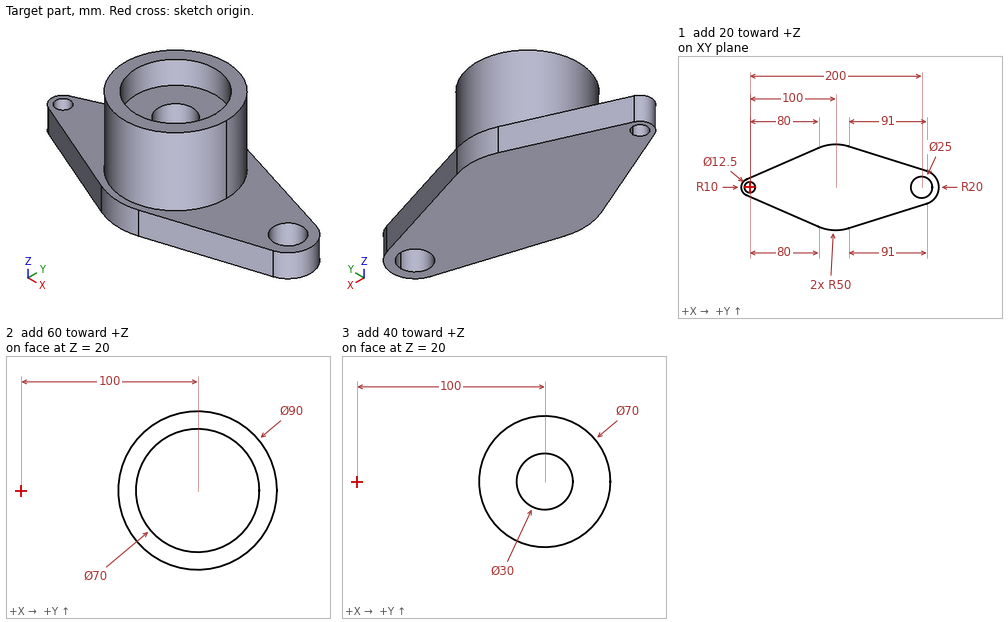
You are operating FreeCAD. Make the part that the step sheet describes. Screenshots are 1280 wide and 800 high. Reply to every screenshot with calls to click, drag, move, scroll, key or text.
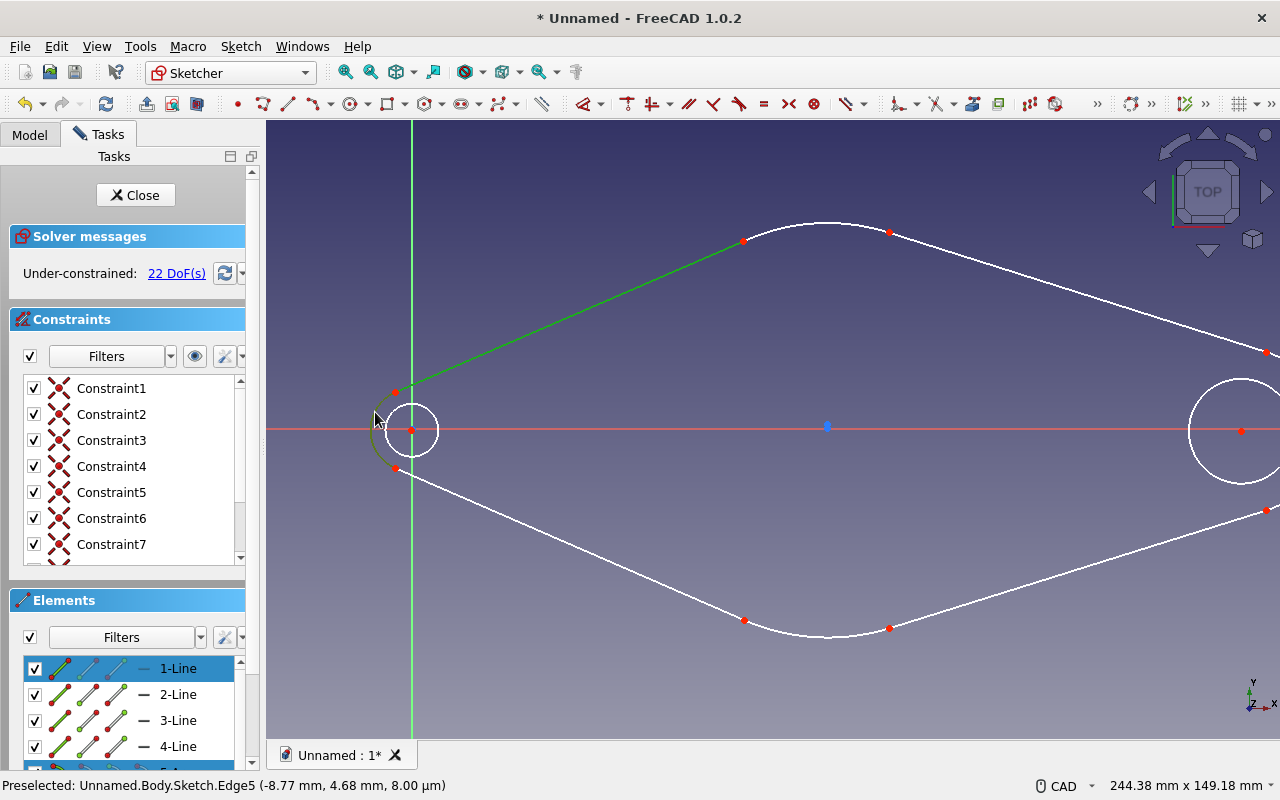
click(739, 104)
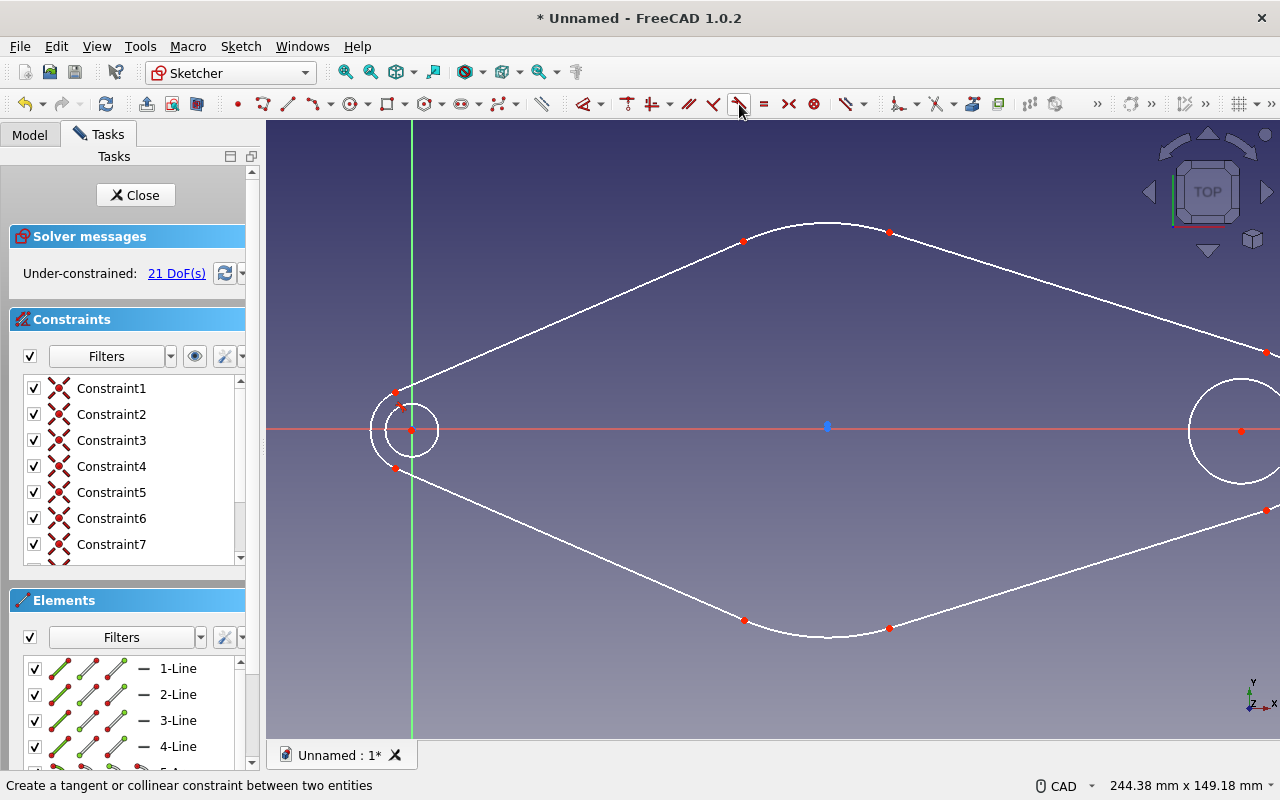
click(500, 514)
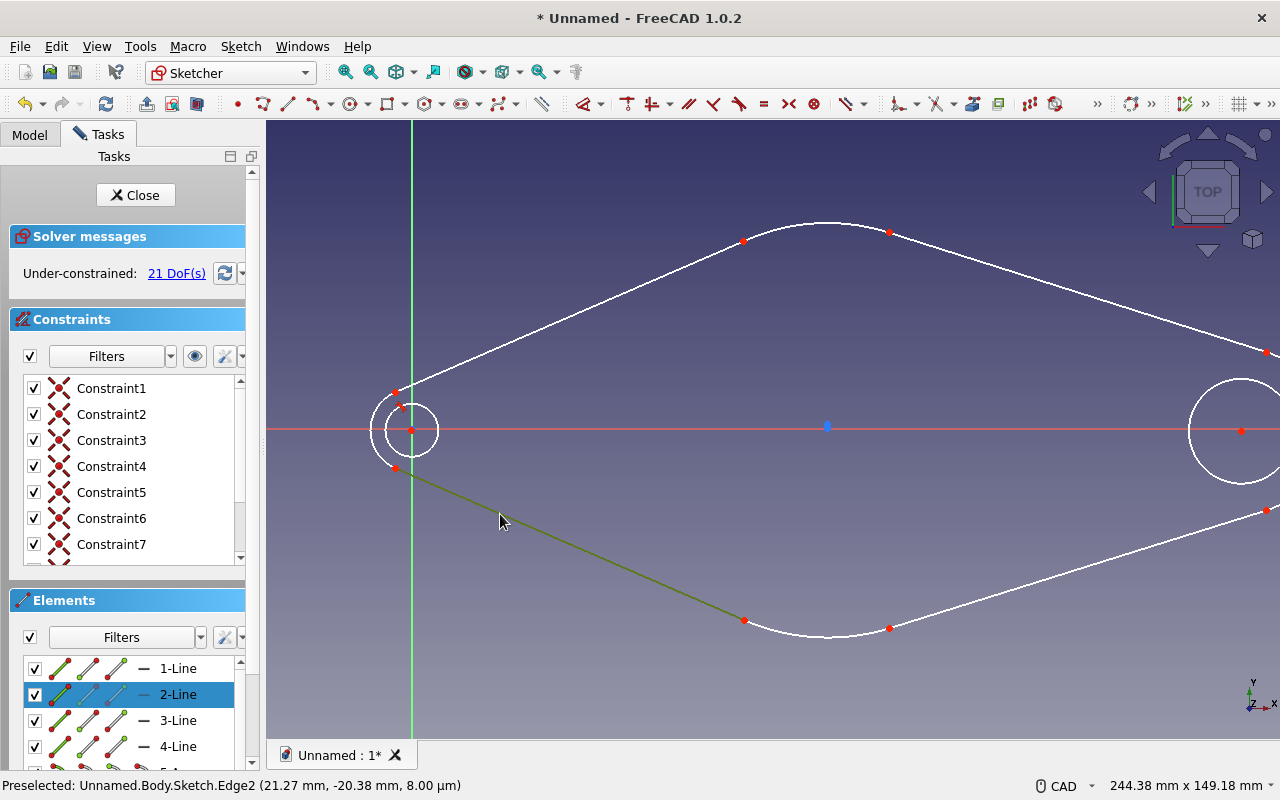
click(375, 412)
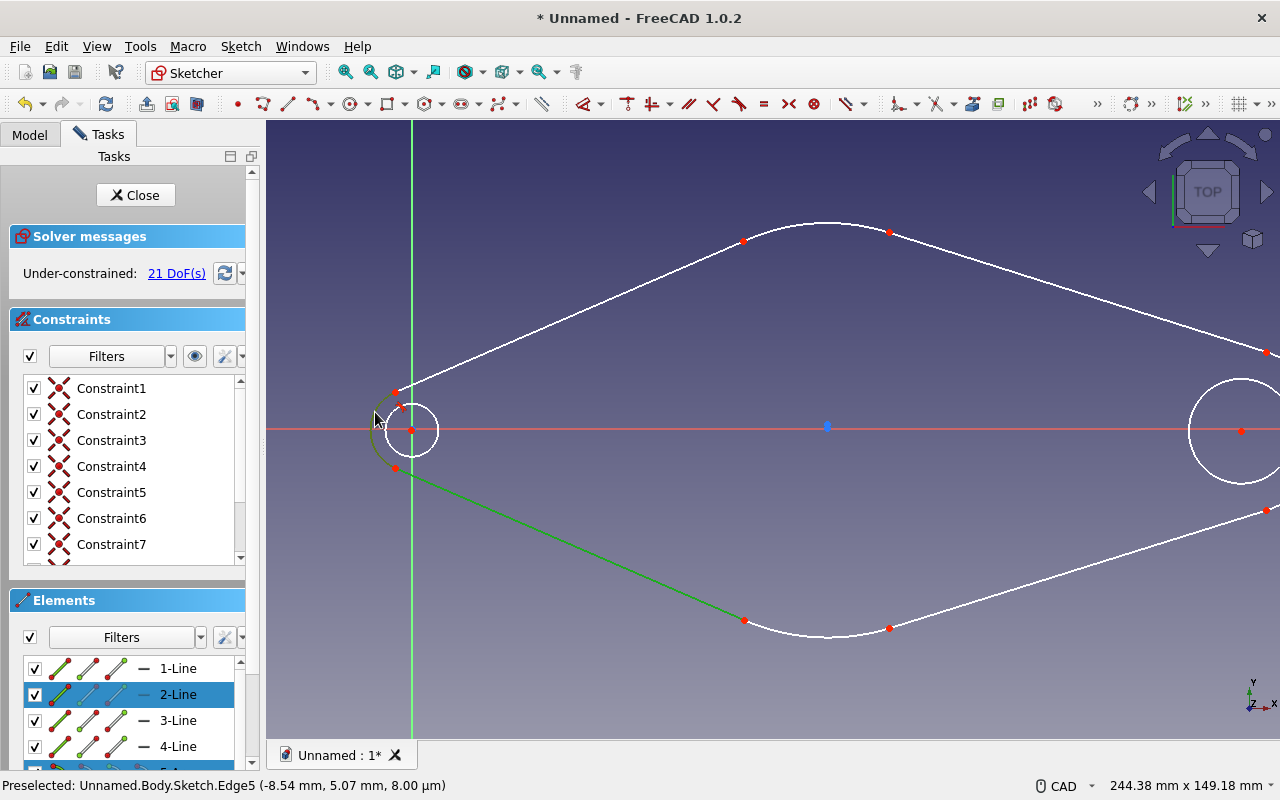
click(739, 104)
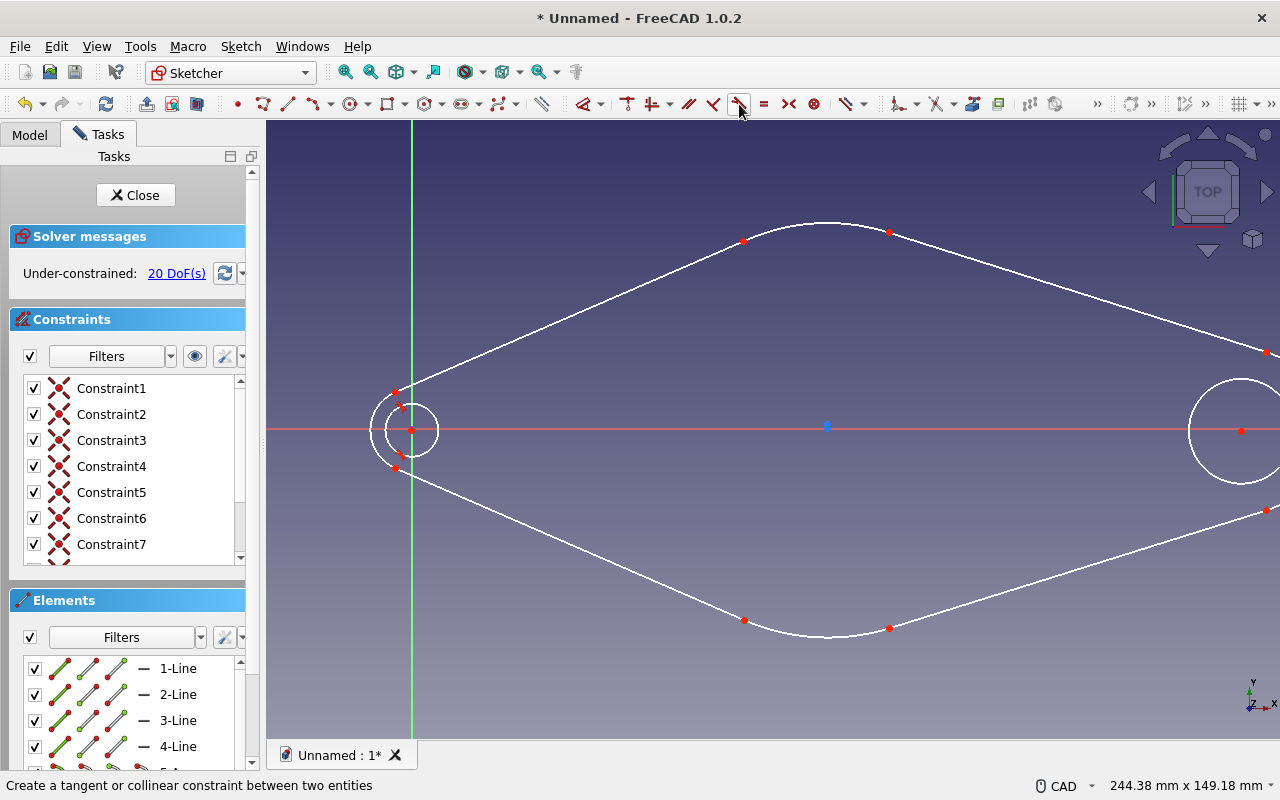
click(1003, 593)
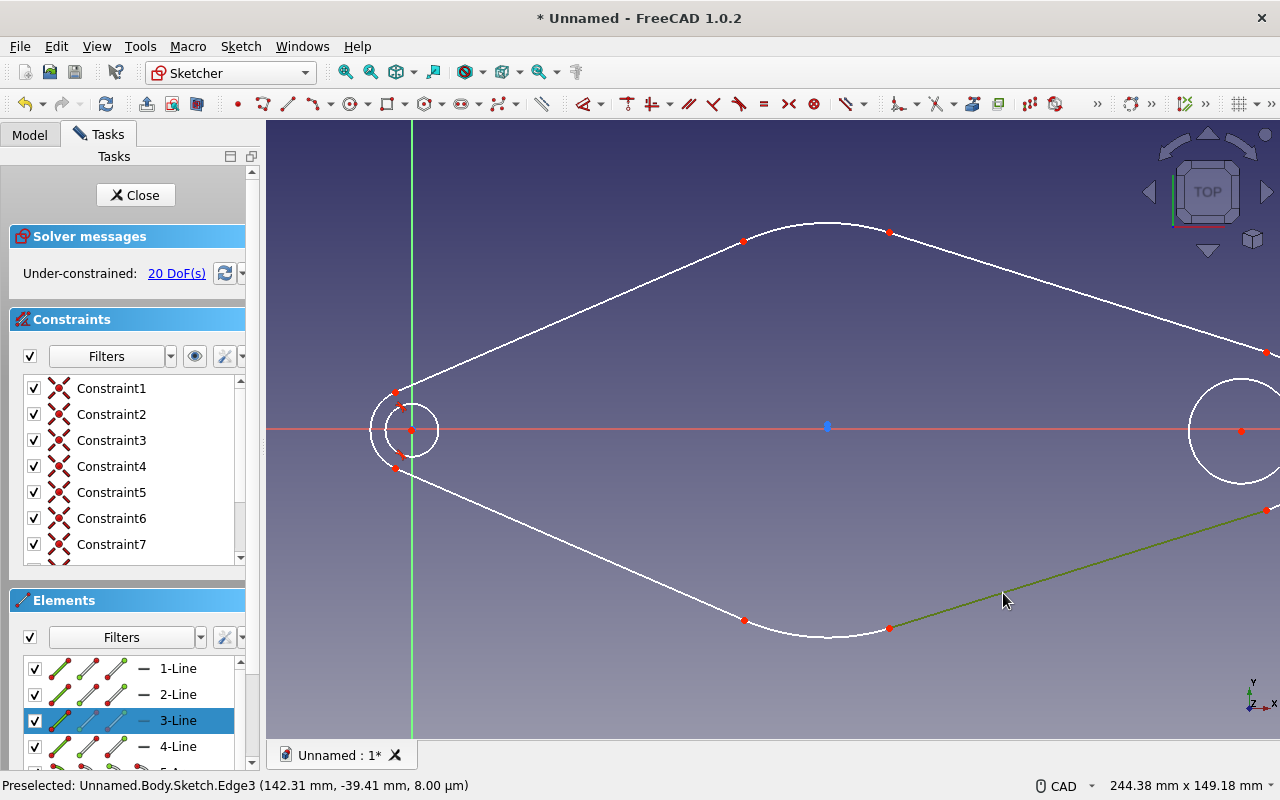
scroll(413, 430, down, 2)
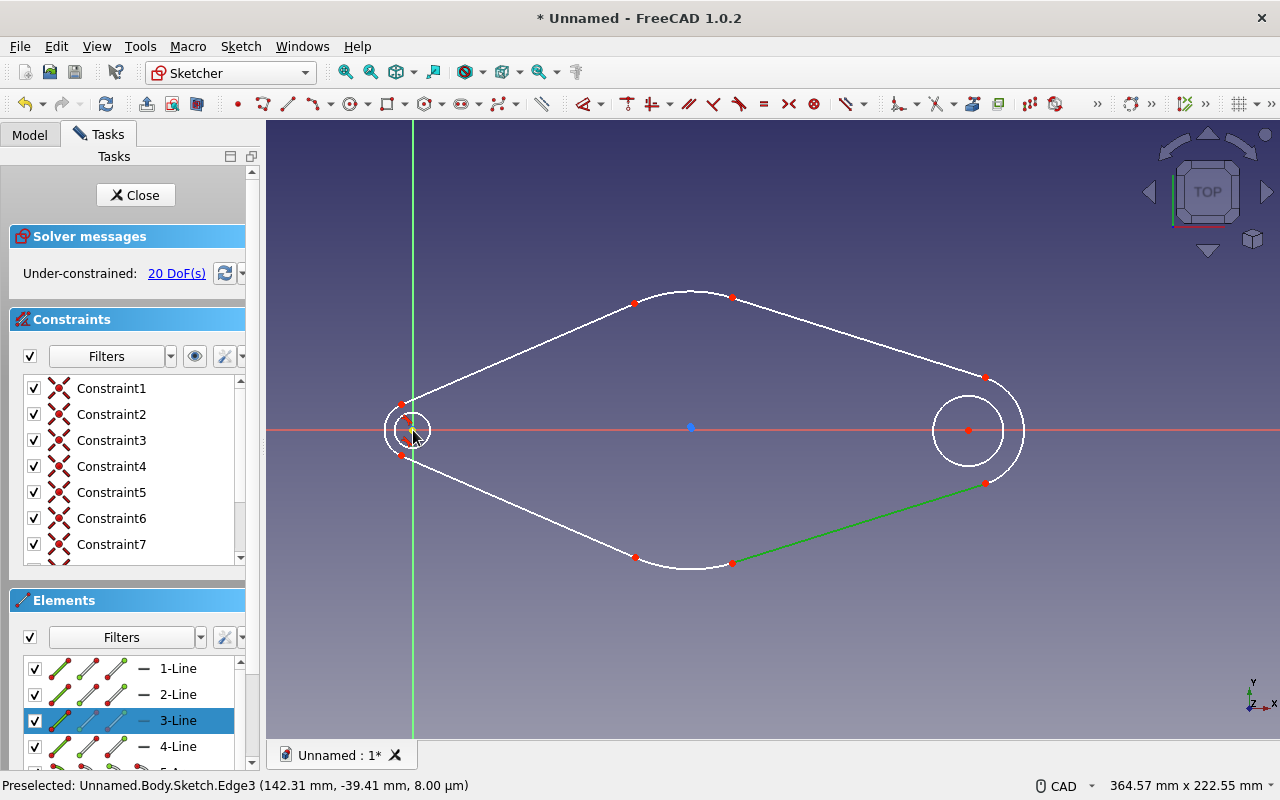
click(1017, 458)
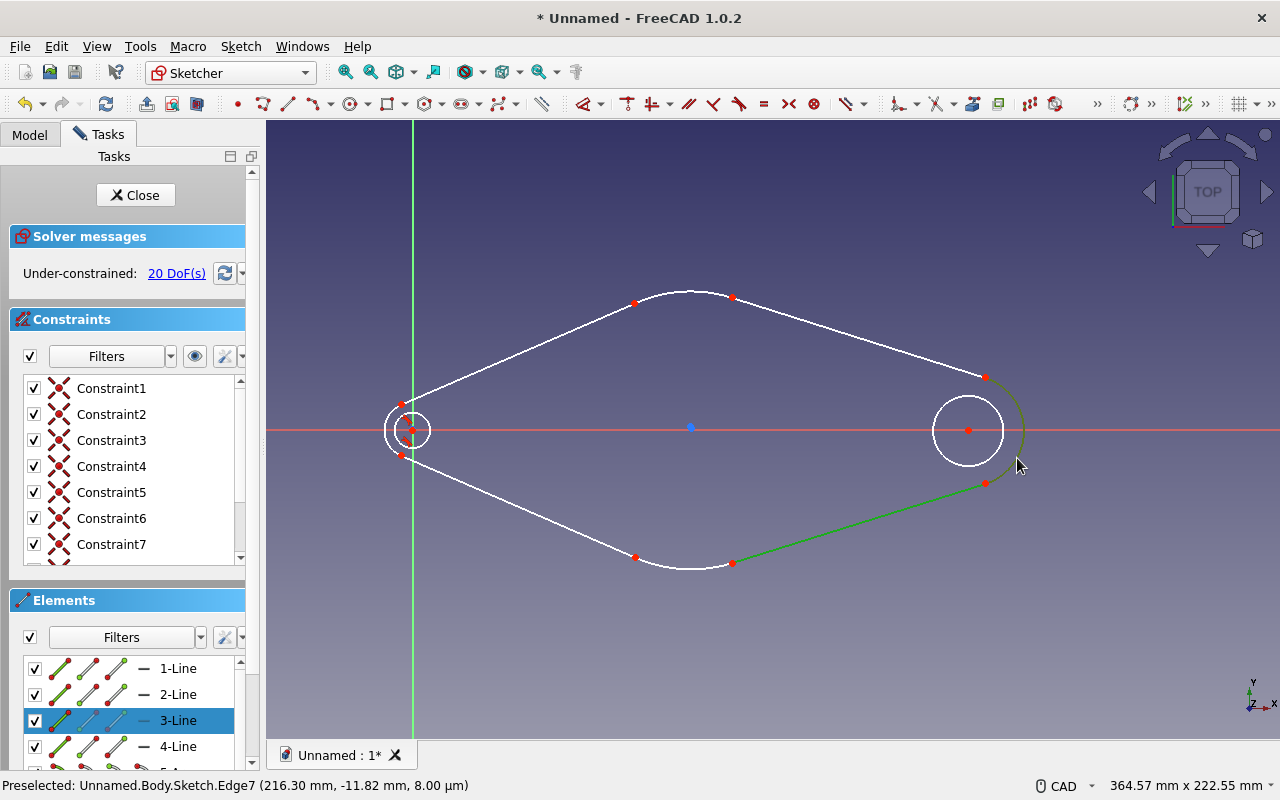
click(739, 104)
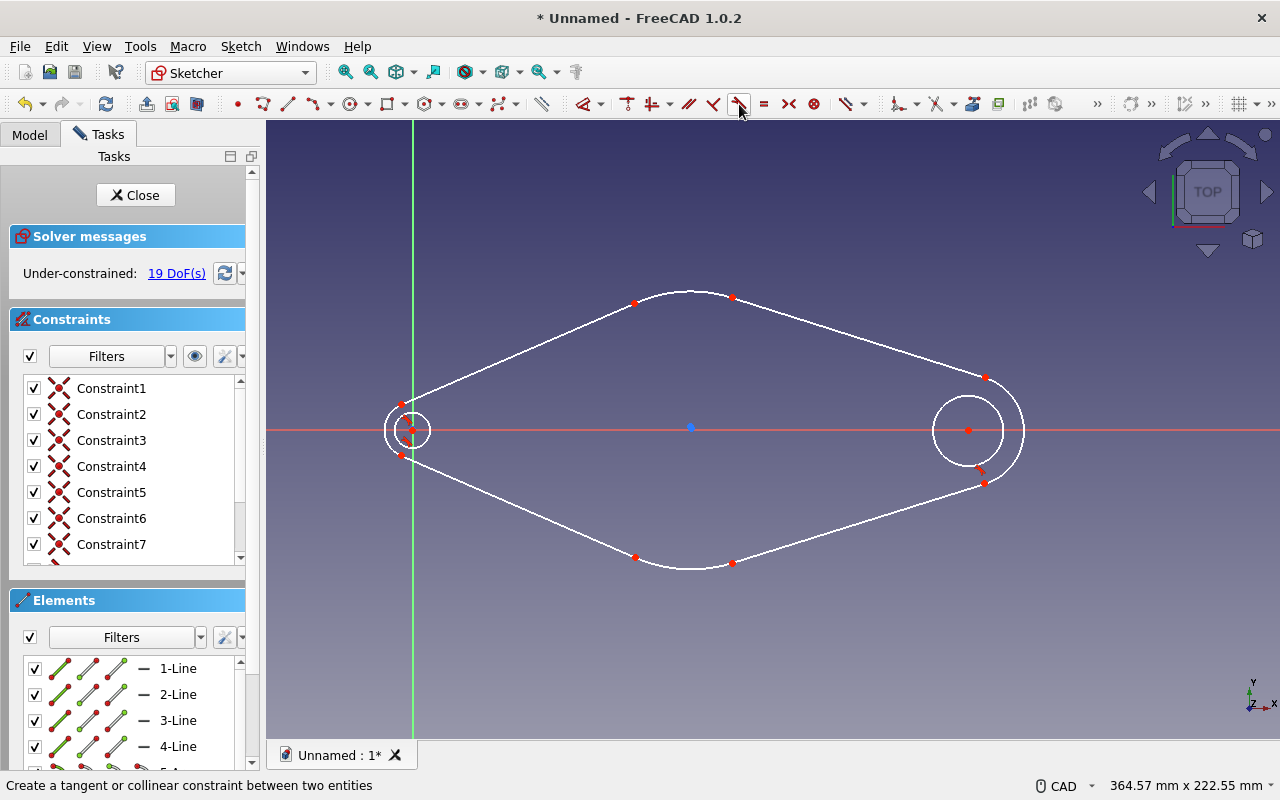
click(909, 354)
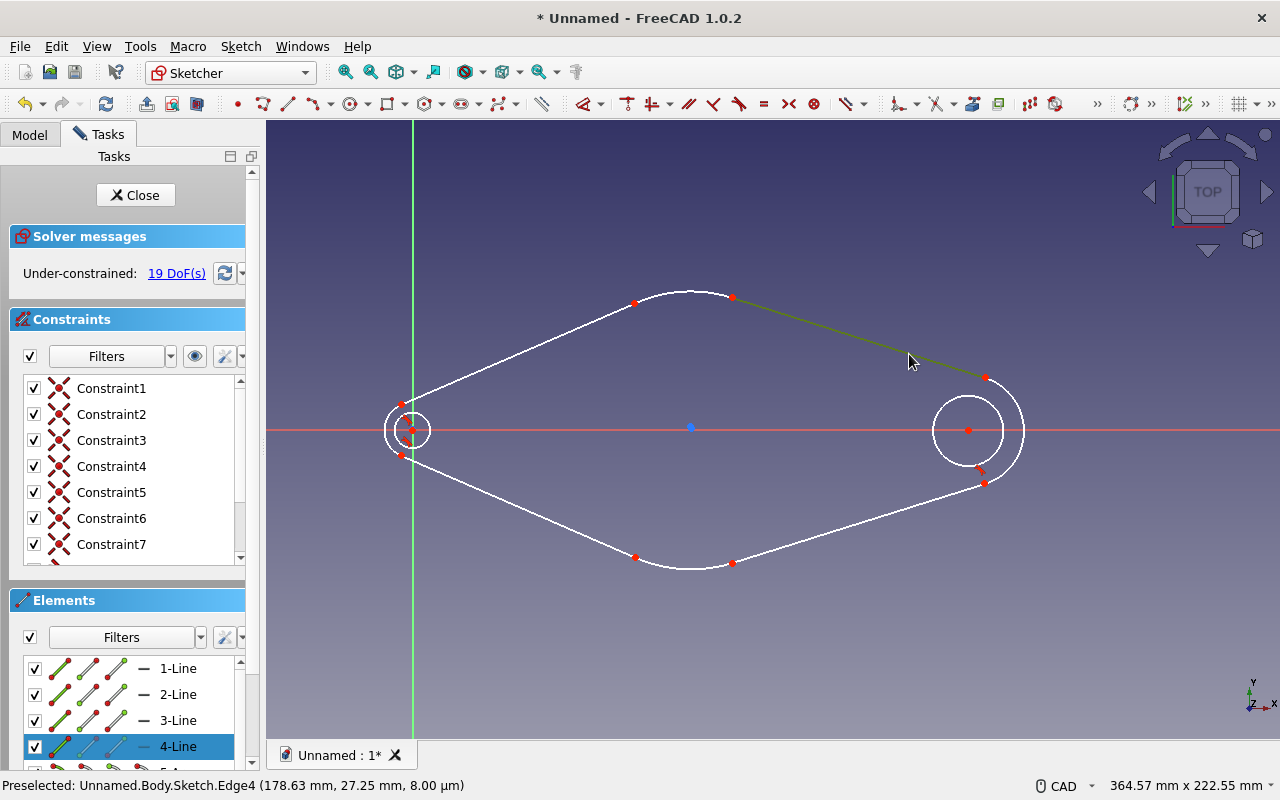
click(1017, 458)